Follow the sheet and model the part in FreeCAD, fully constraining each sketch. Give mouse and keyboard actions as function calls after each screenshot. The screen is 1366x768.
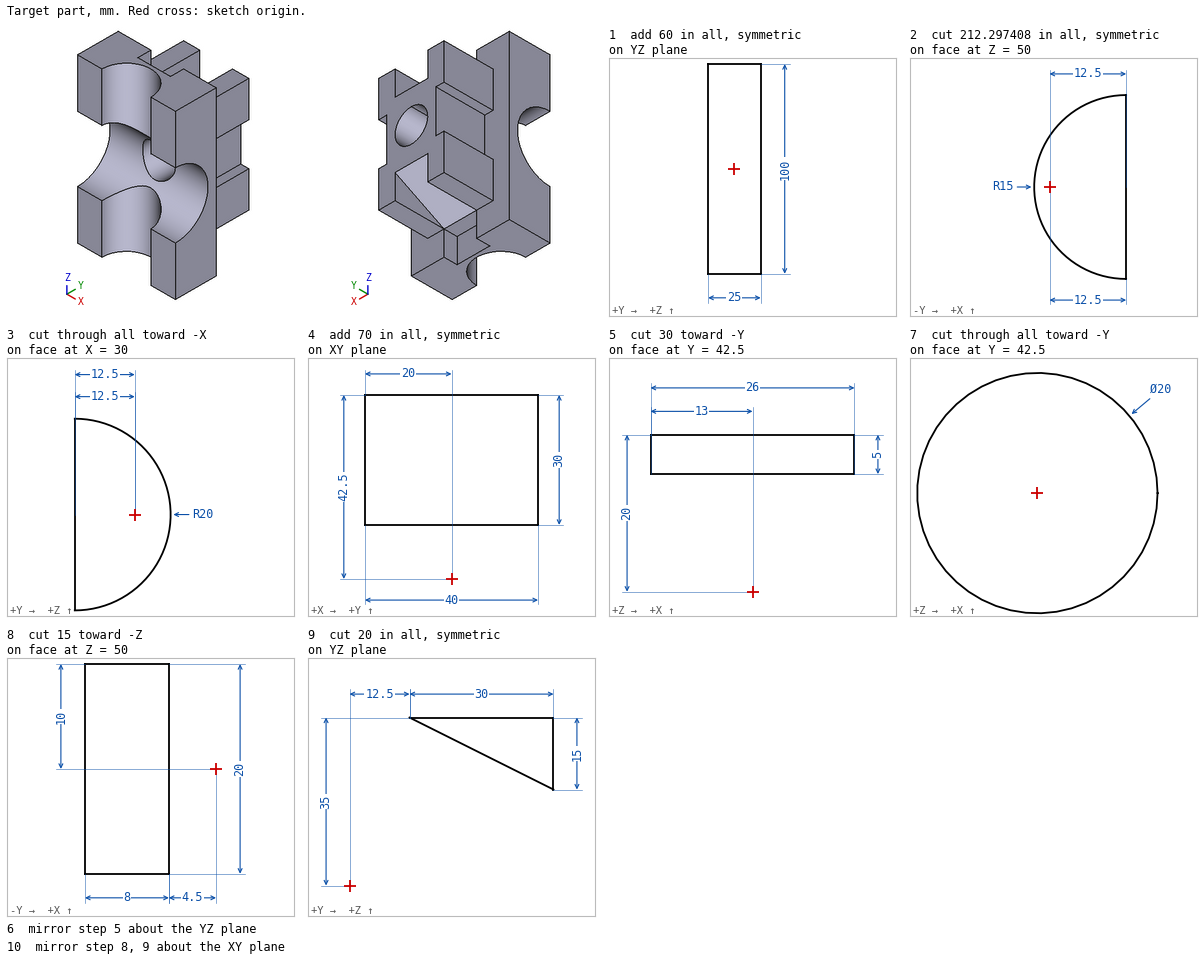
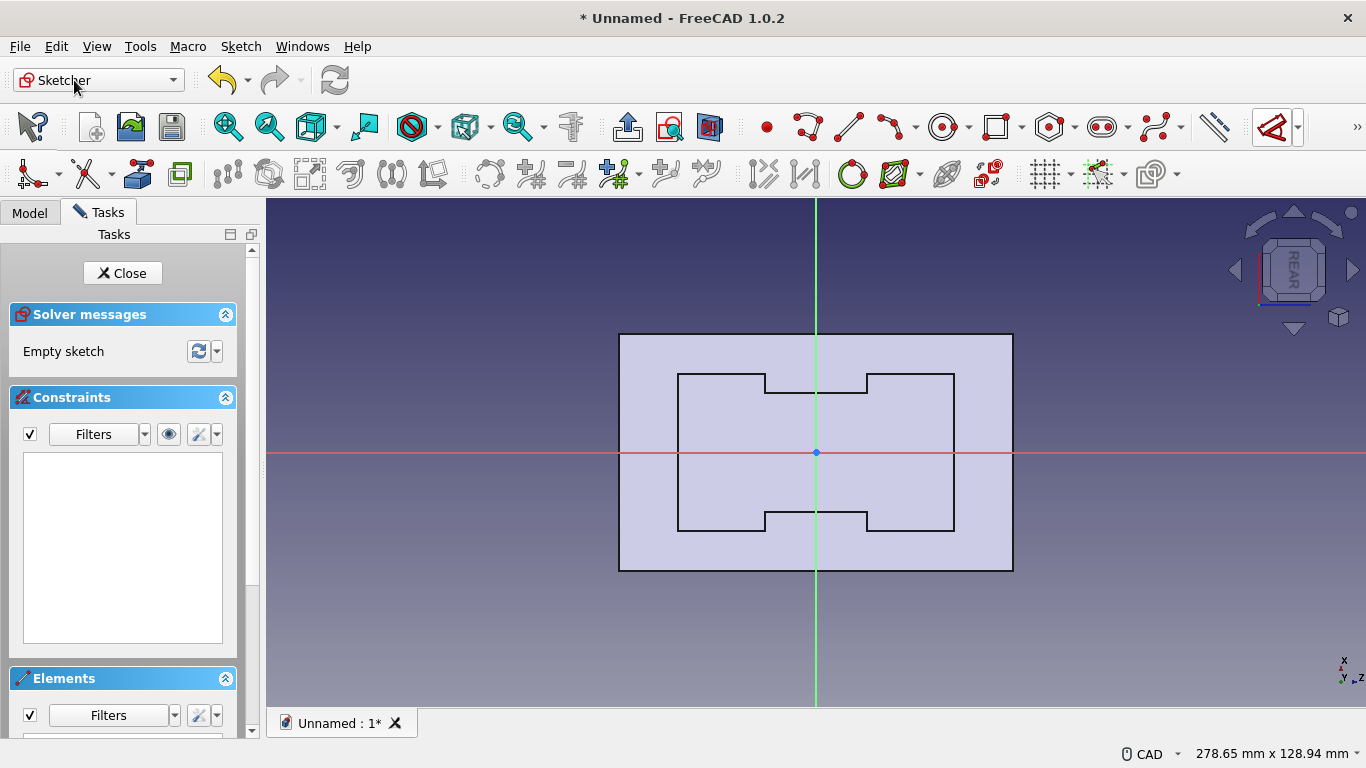
scroll(838, 453, up, 7)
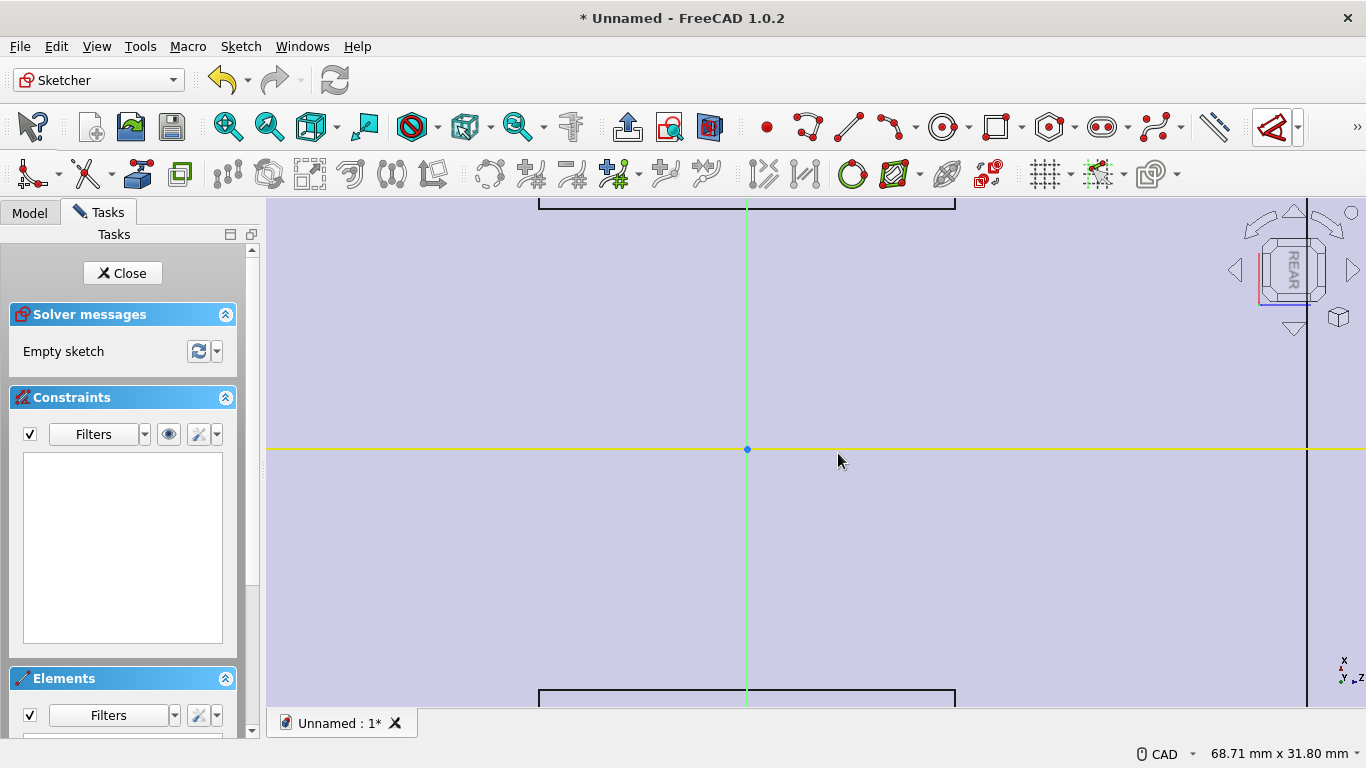
click(942, 128)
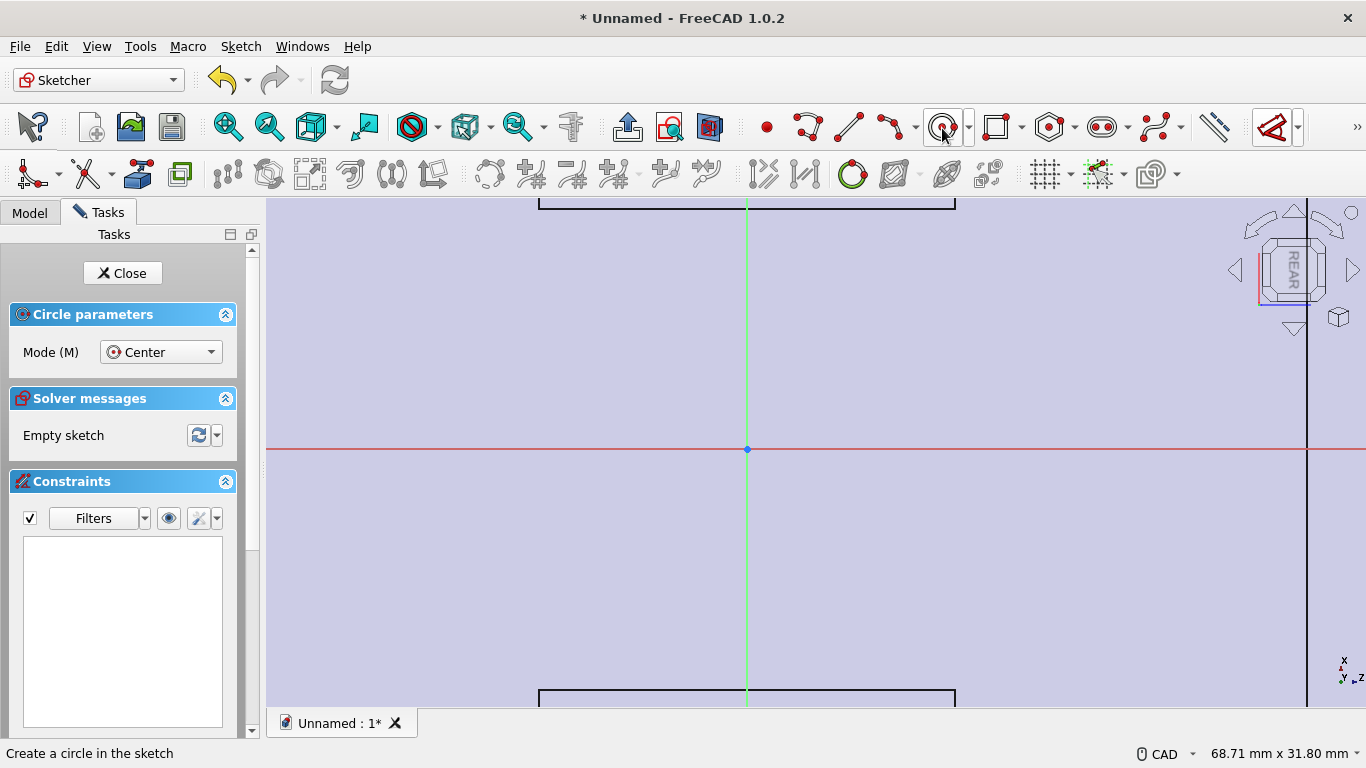
click(747, 449)
move(860, 336)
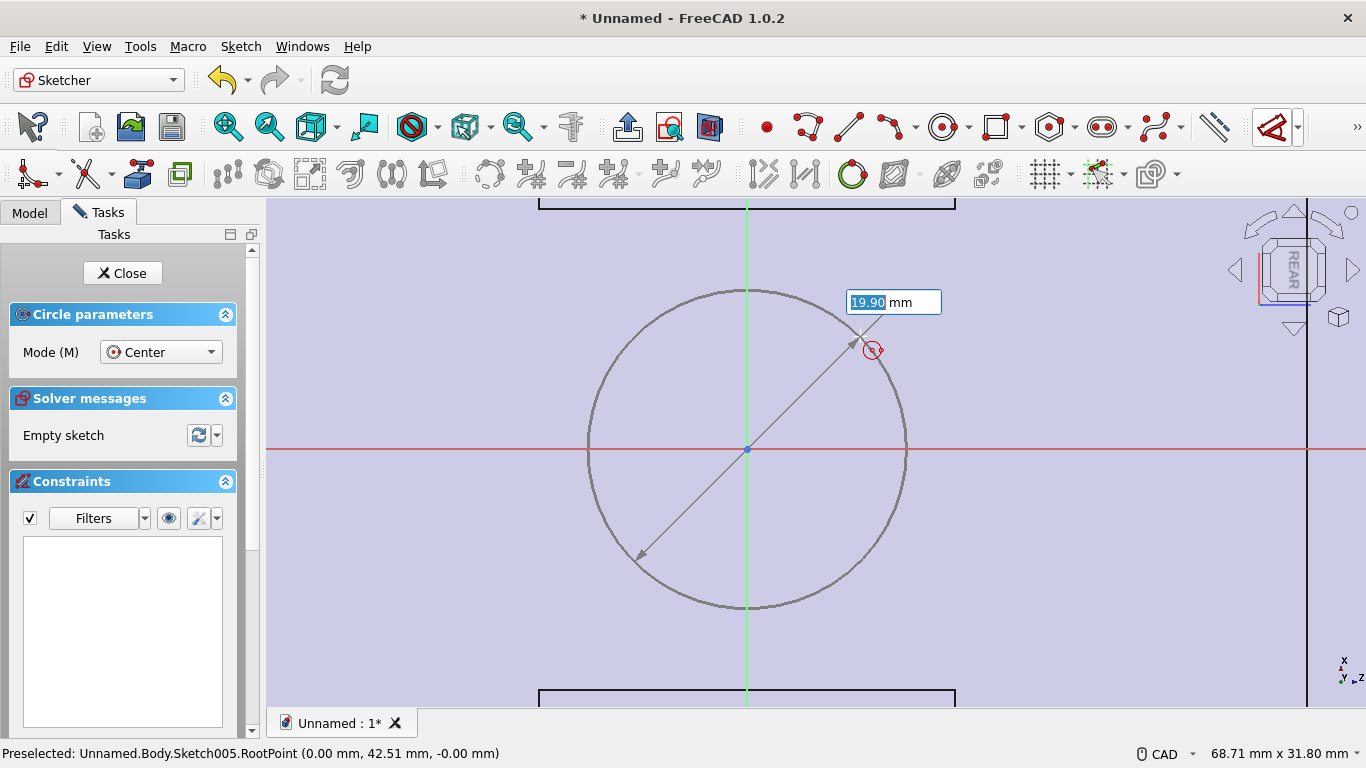
text(20)
key(Return)
key(Escape)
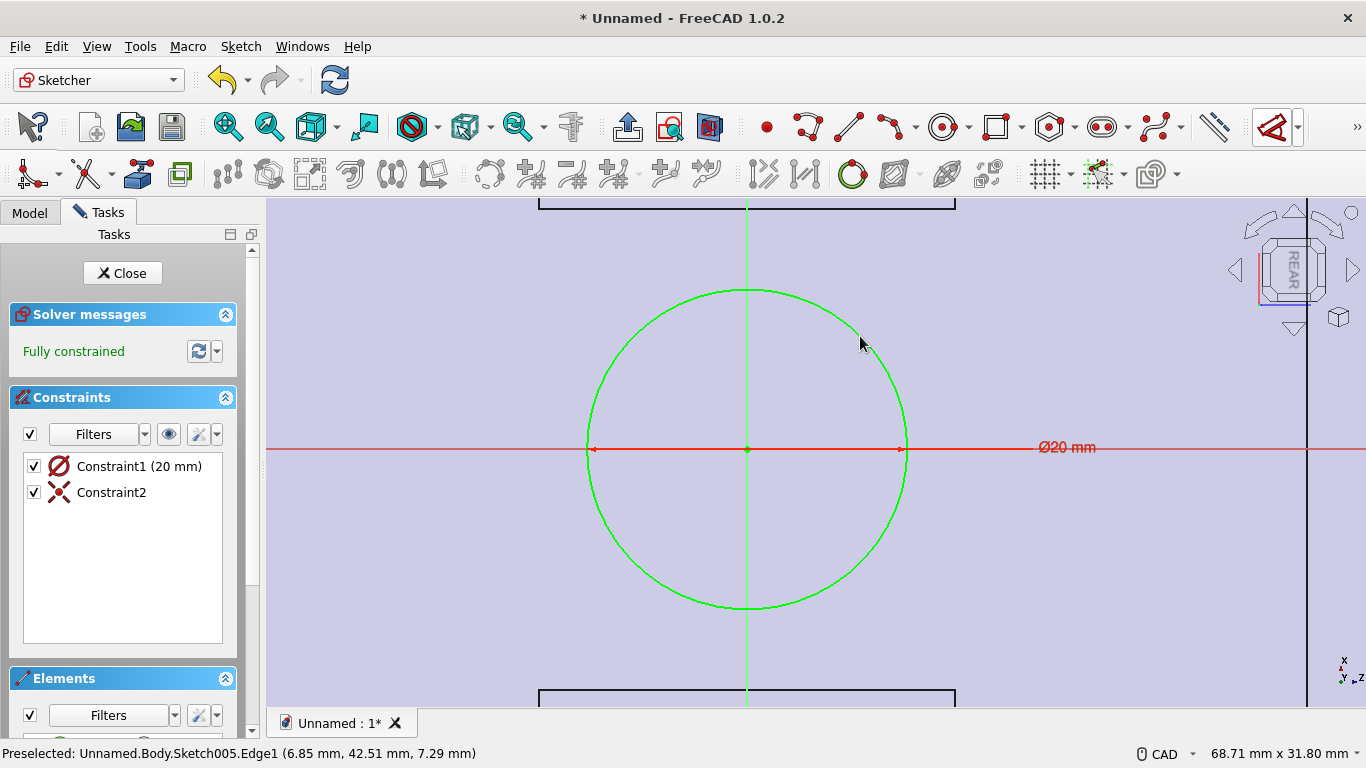
click(123, 273)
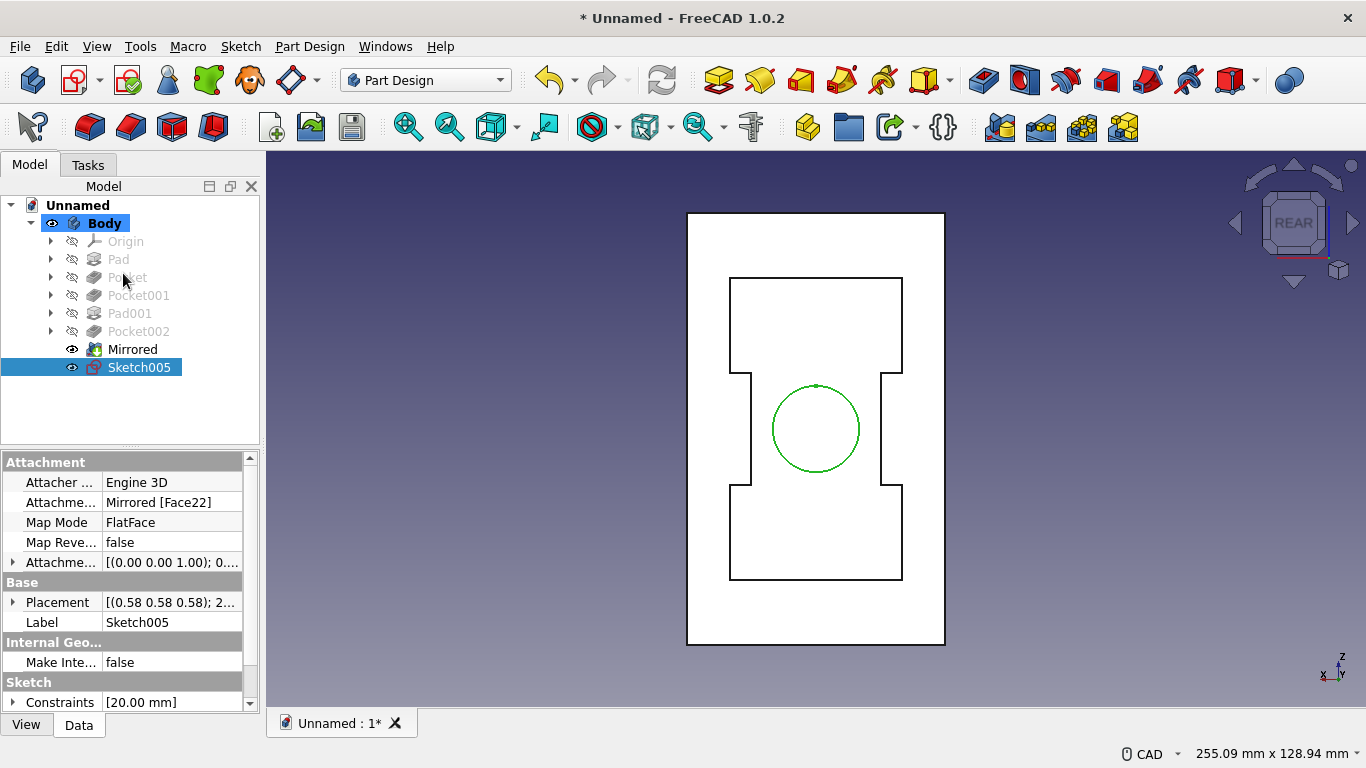
click(984, 80)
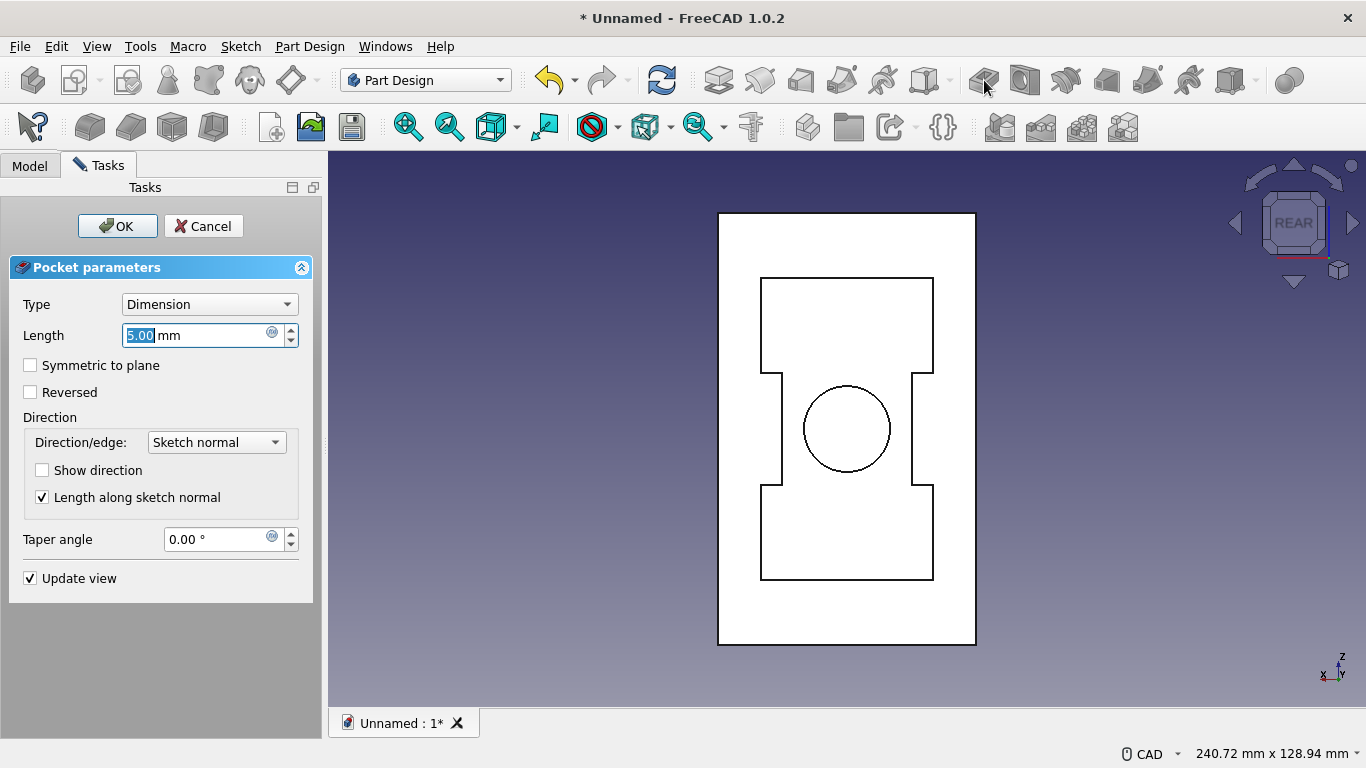
click(210, 304)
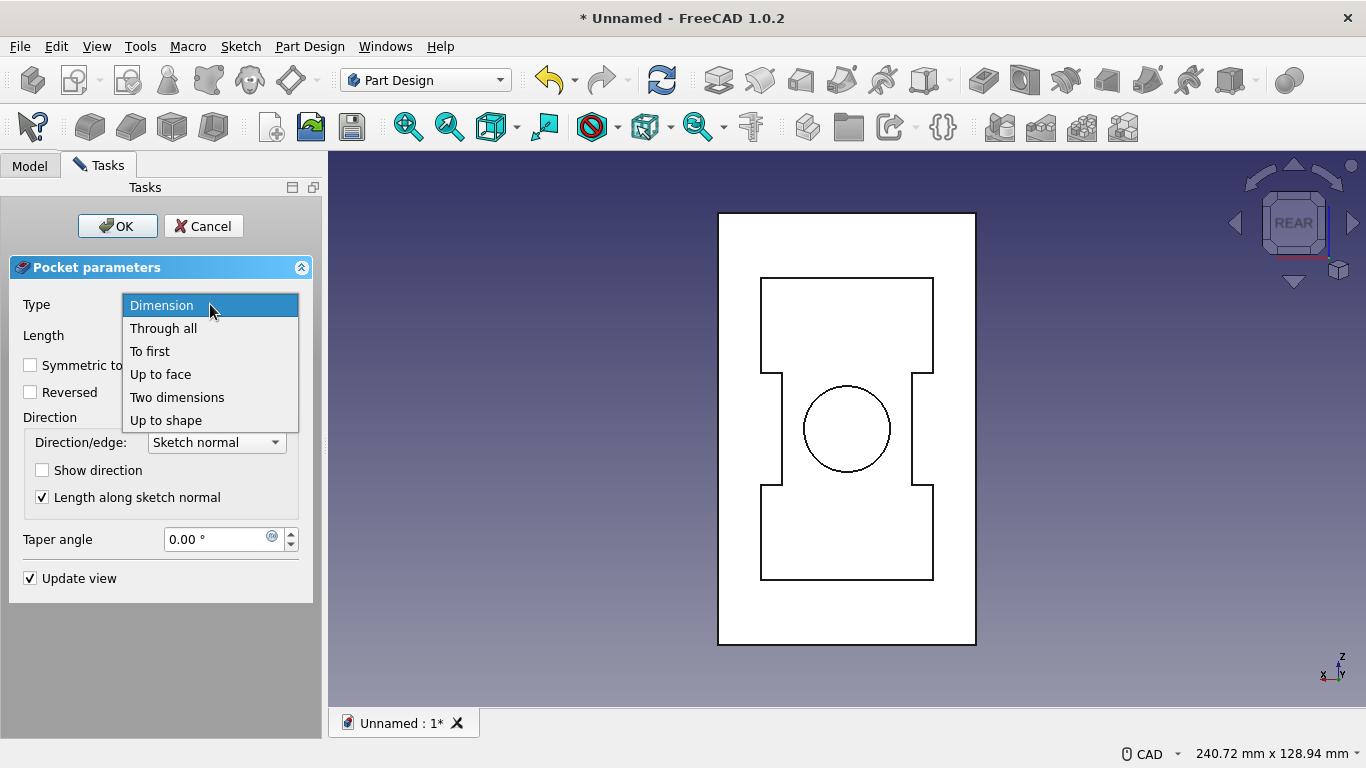
click(208, 328)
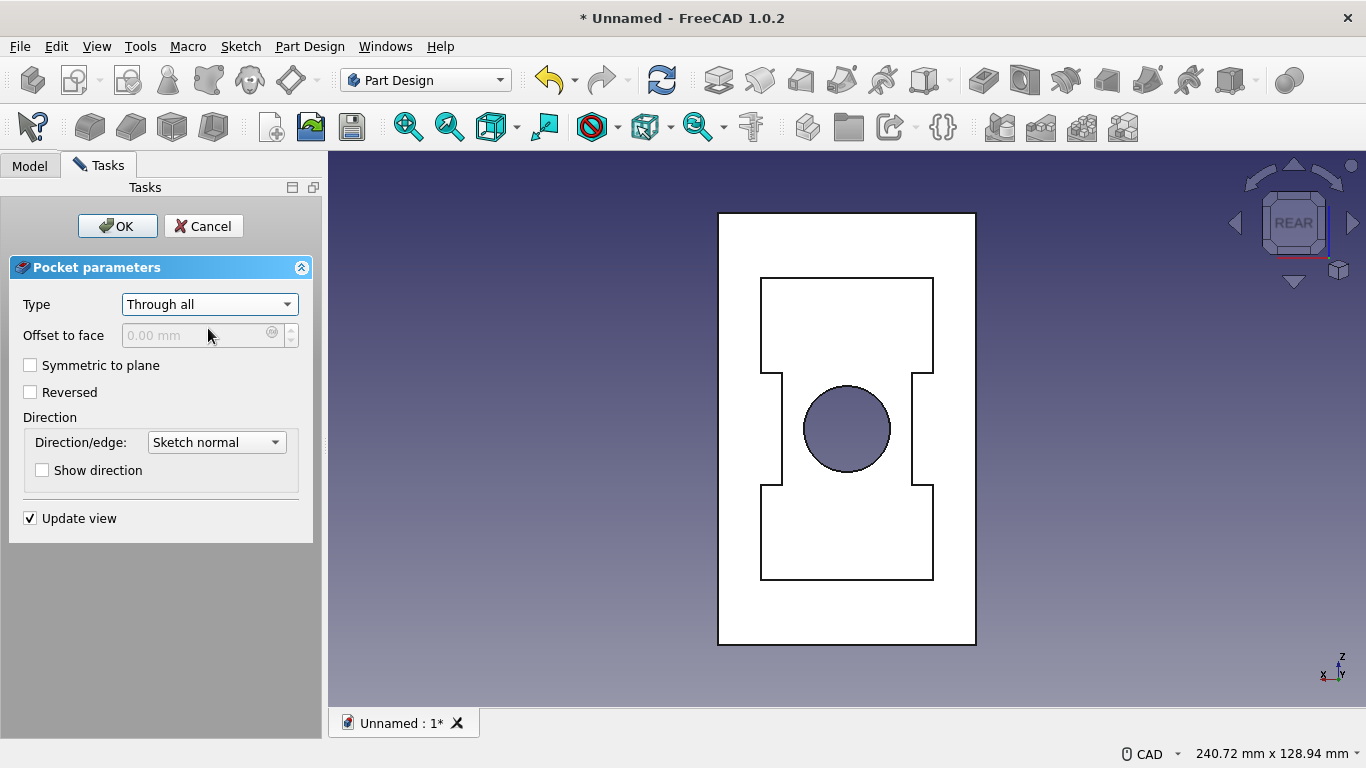
click(118, 226)